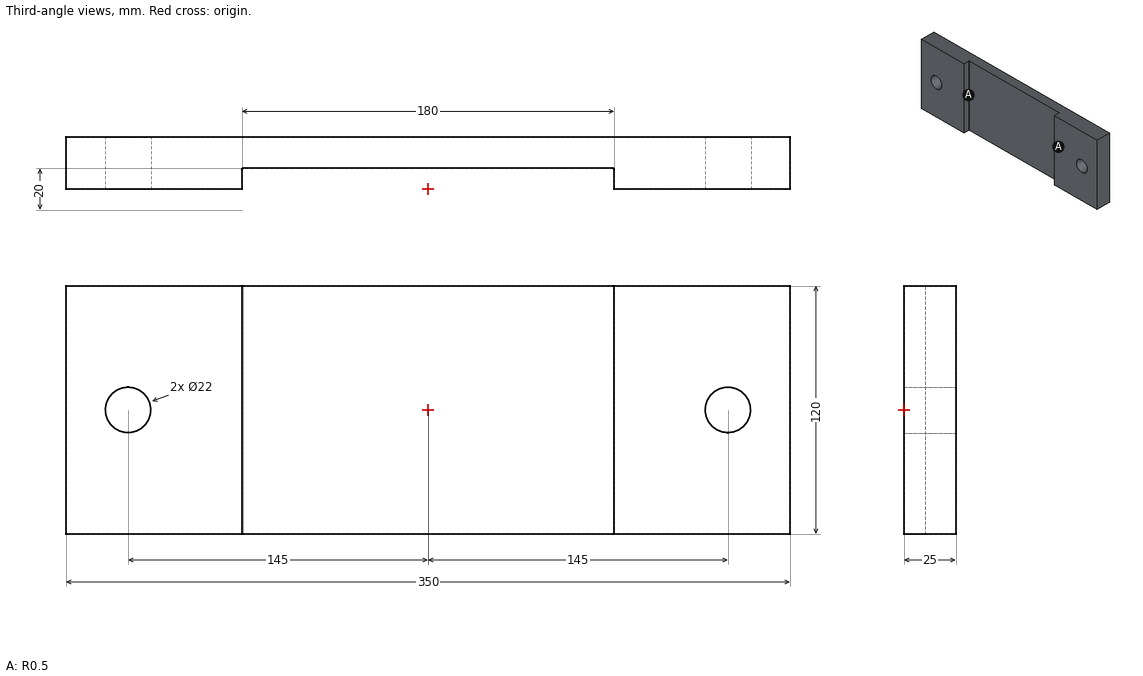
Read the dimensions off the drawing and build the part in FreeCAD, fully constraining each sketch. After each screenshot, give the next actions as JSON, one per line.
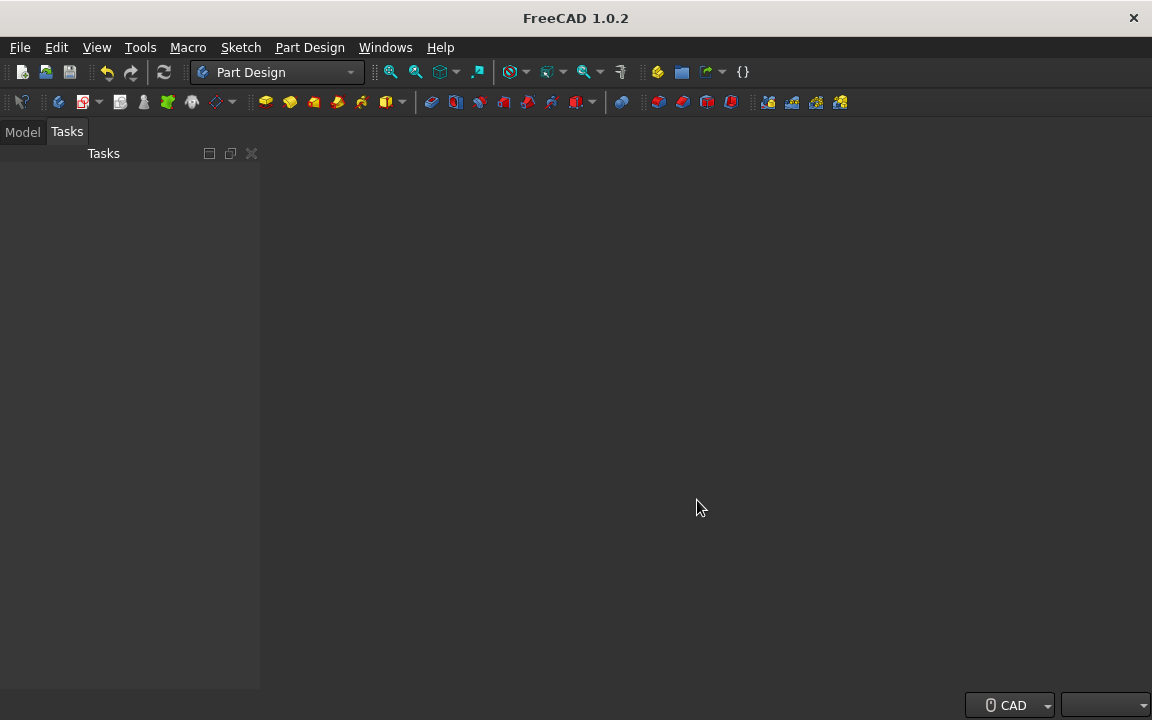
{"action": "left_click", "coordinate": [22, 72]}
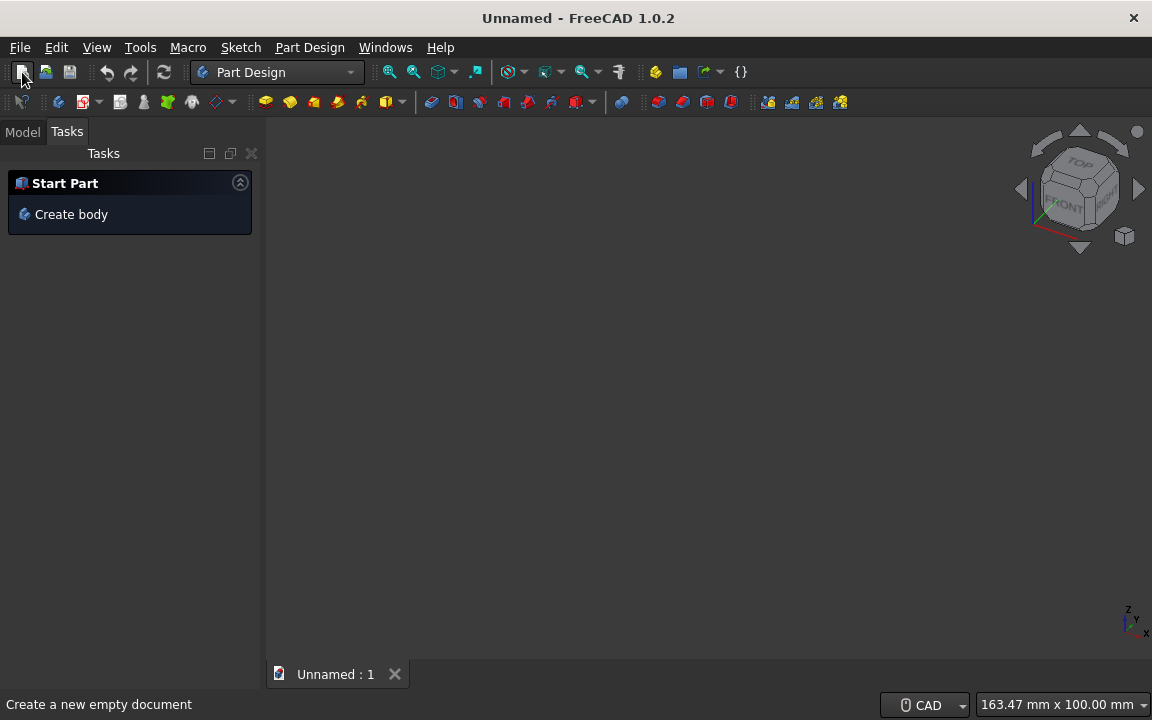
{"action": "left_click", "coordinate": [84, 102]}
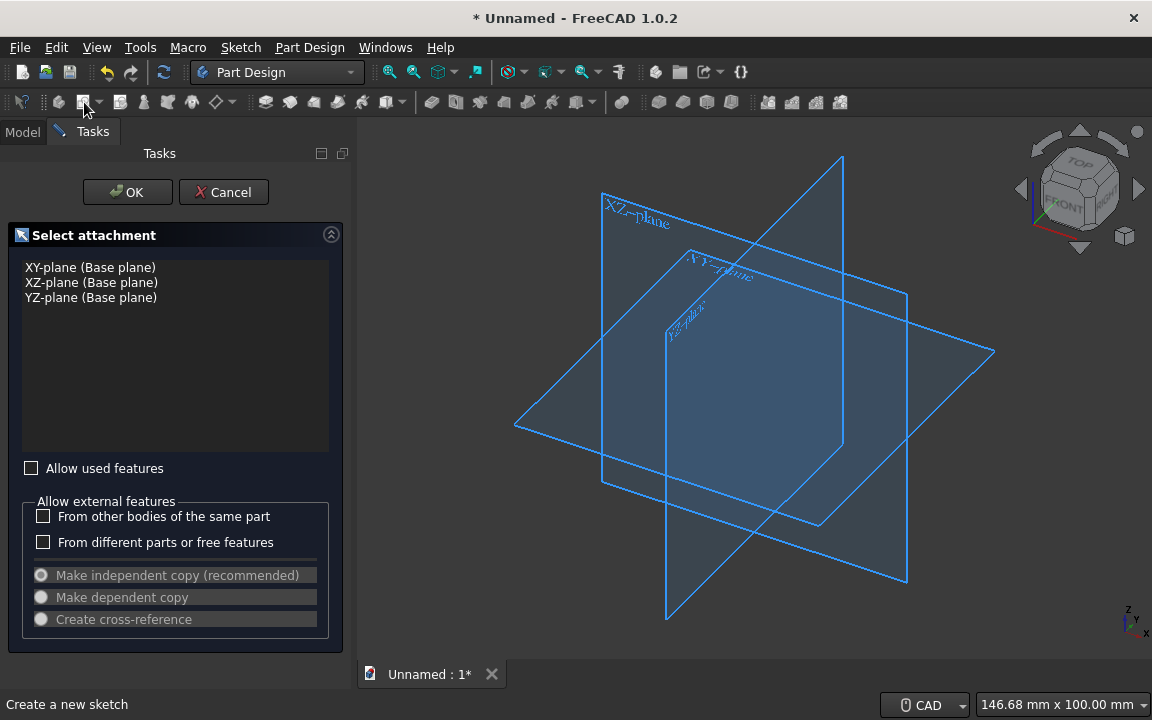
{"action": "left_click", "coordinate": [82, 282]}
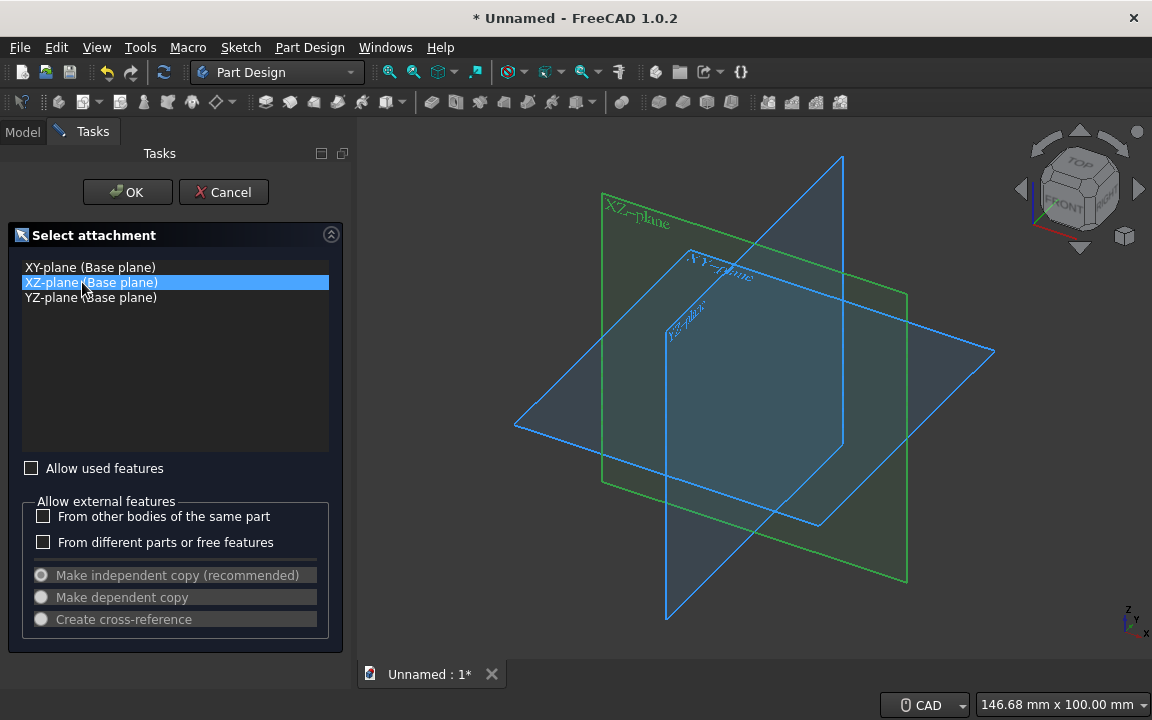
{"action": "left_click", "coordinate": [128, 192]}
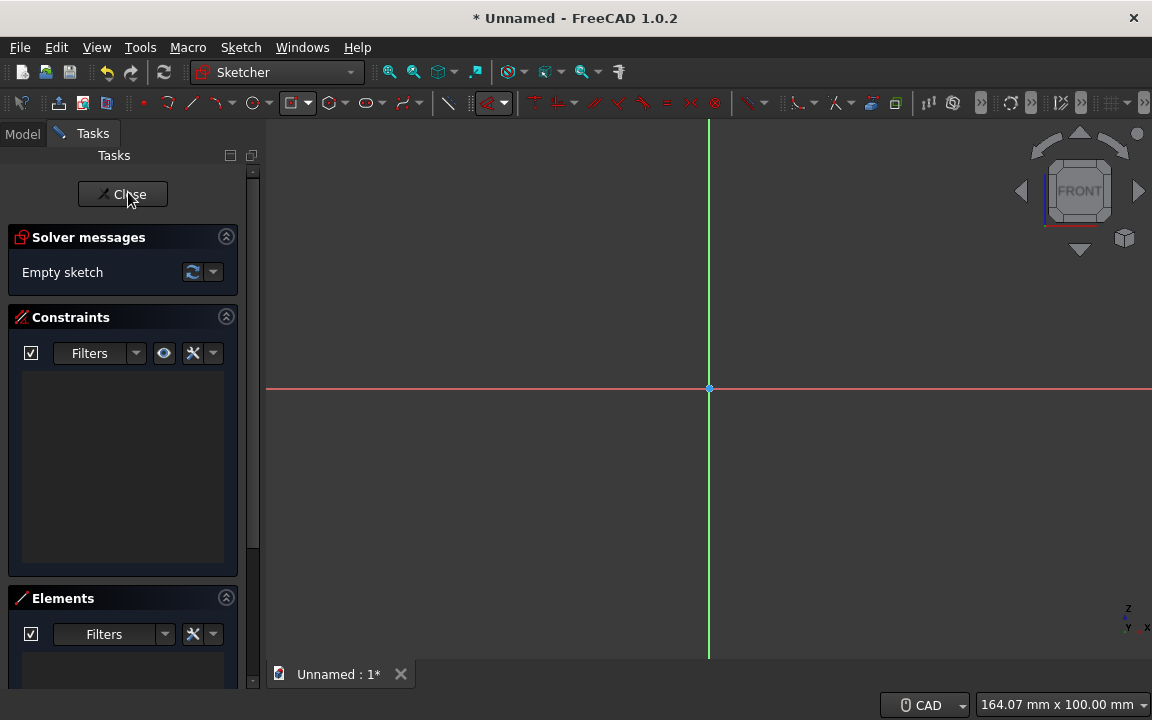
{"action": "scroll", "coordinate": [618, 389], "scroll_direction": "down", "scroll_amount": 7}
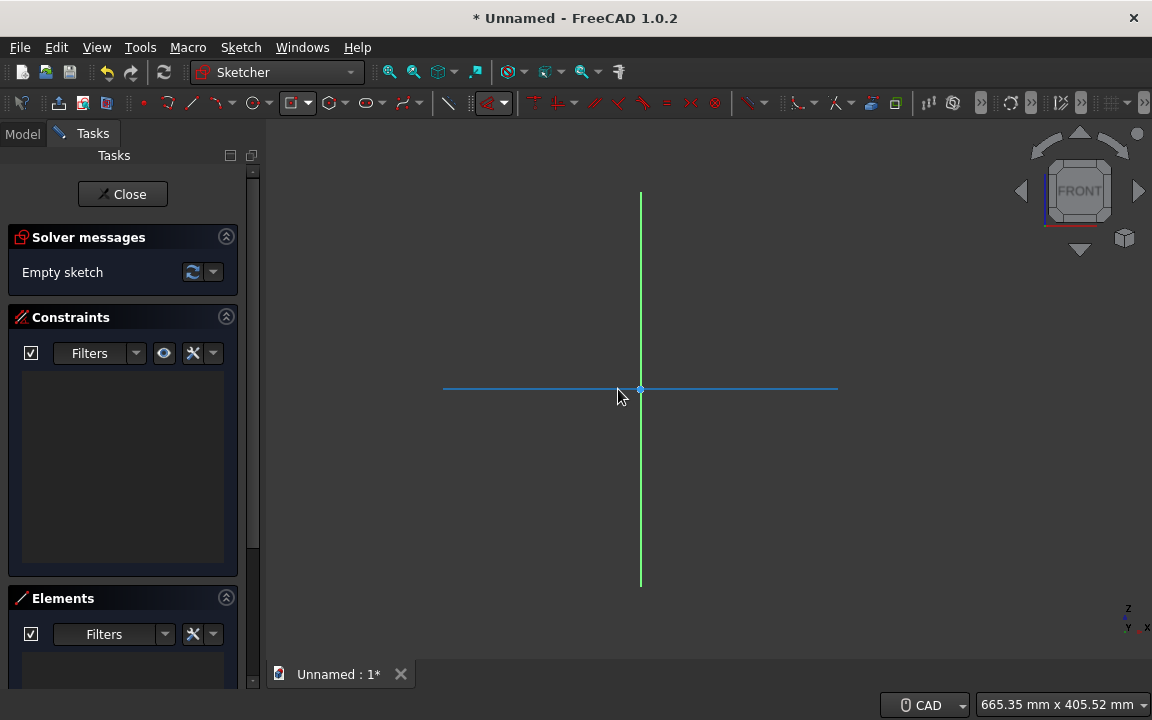
{"action": "left_click", "coordinate": [292, 104]}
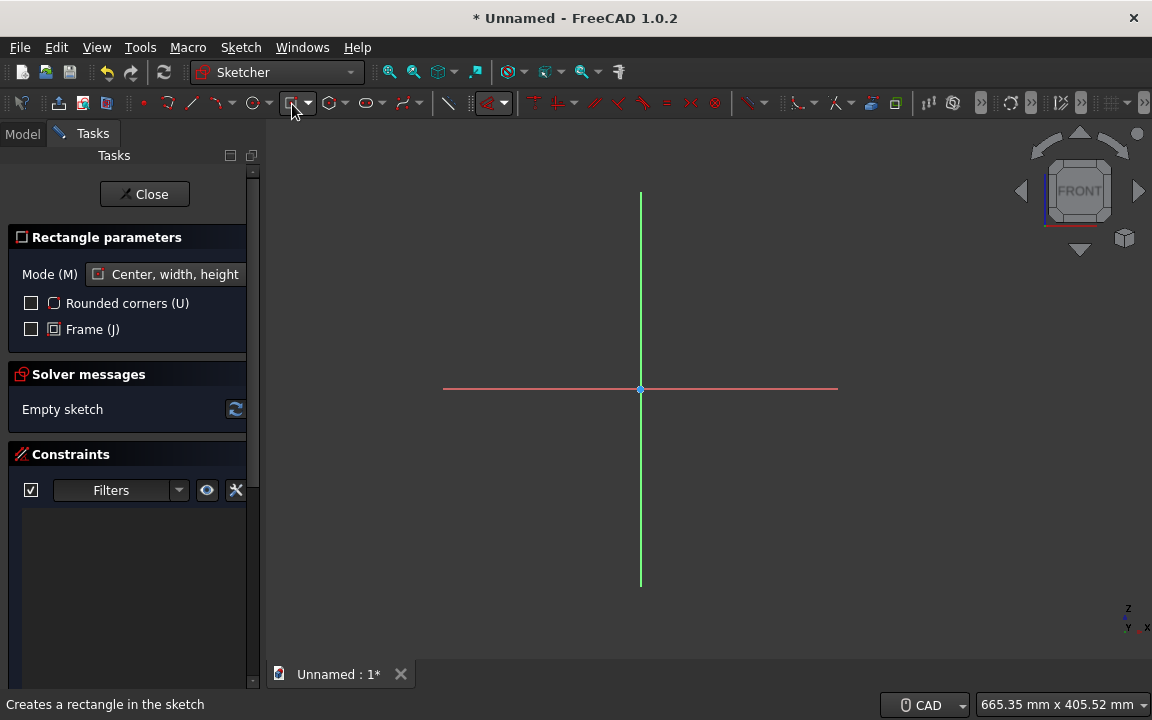
{"action": "left_click", "coordinate": [641, 389]}
{"action": "mouse_move", "coordinate": [874, 309]}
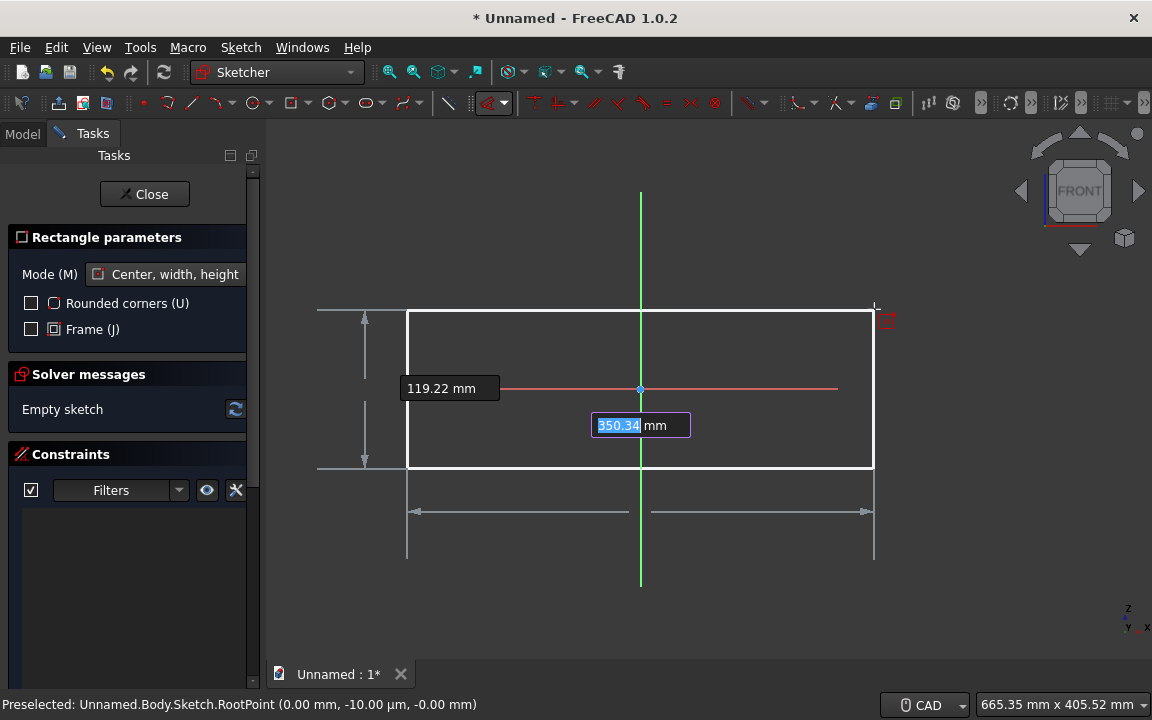
{"action": "type", "text": "350"}
{"action": "key", "text": "Tab"}
{"action": "type", "text": "120"}
{"action": "key", "text": "Return"}
{"action": "key", "text": "Escape"}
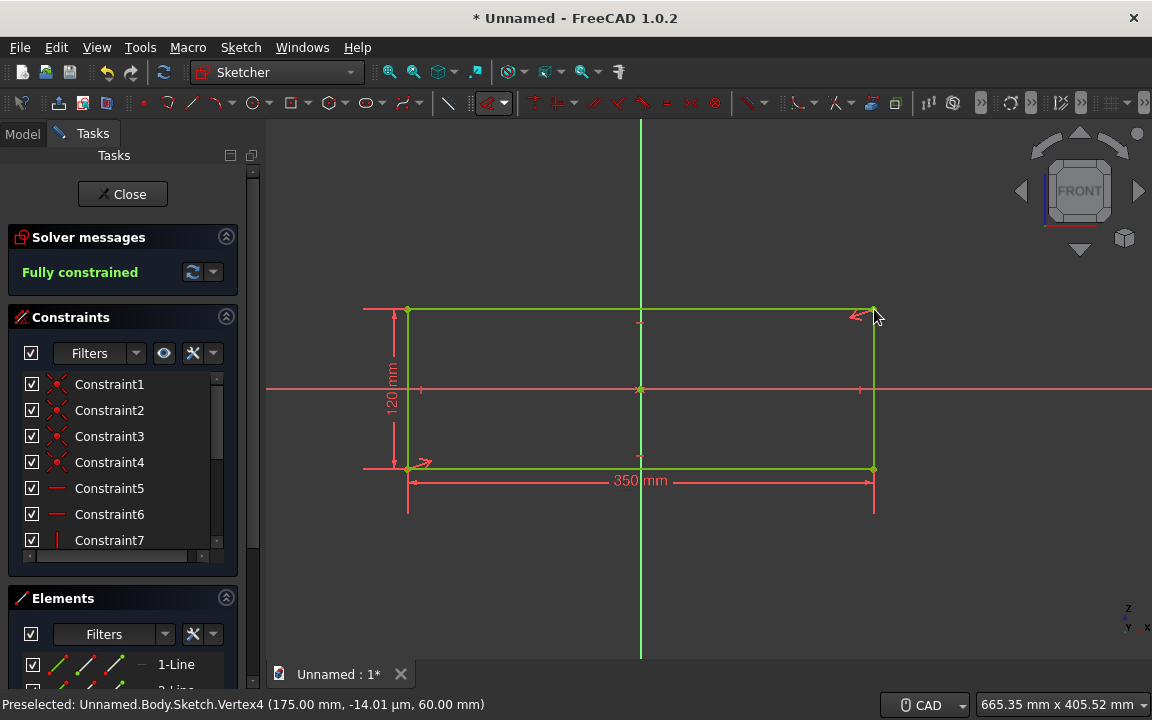
{"action": "left_click", "coordinate": [123, 194]}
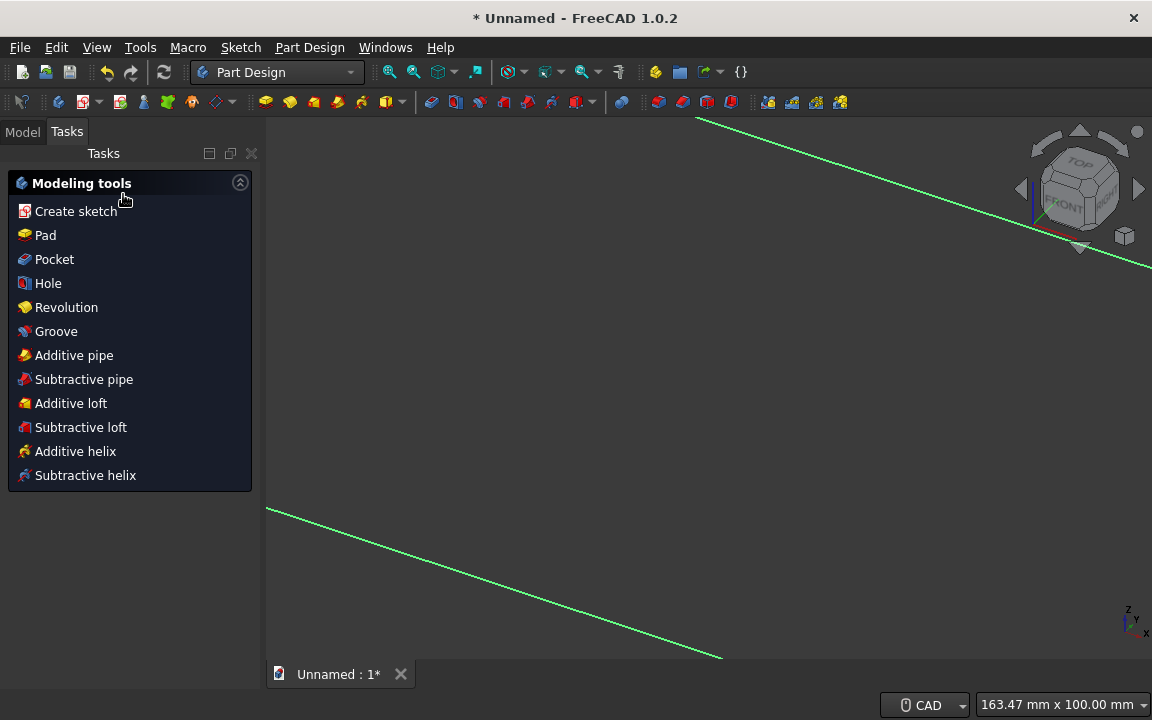
{"action": "left_click", "coordinate": [266, 102]}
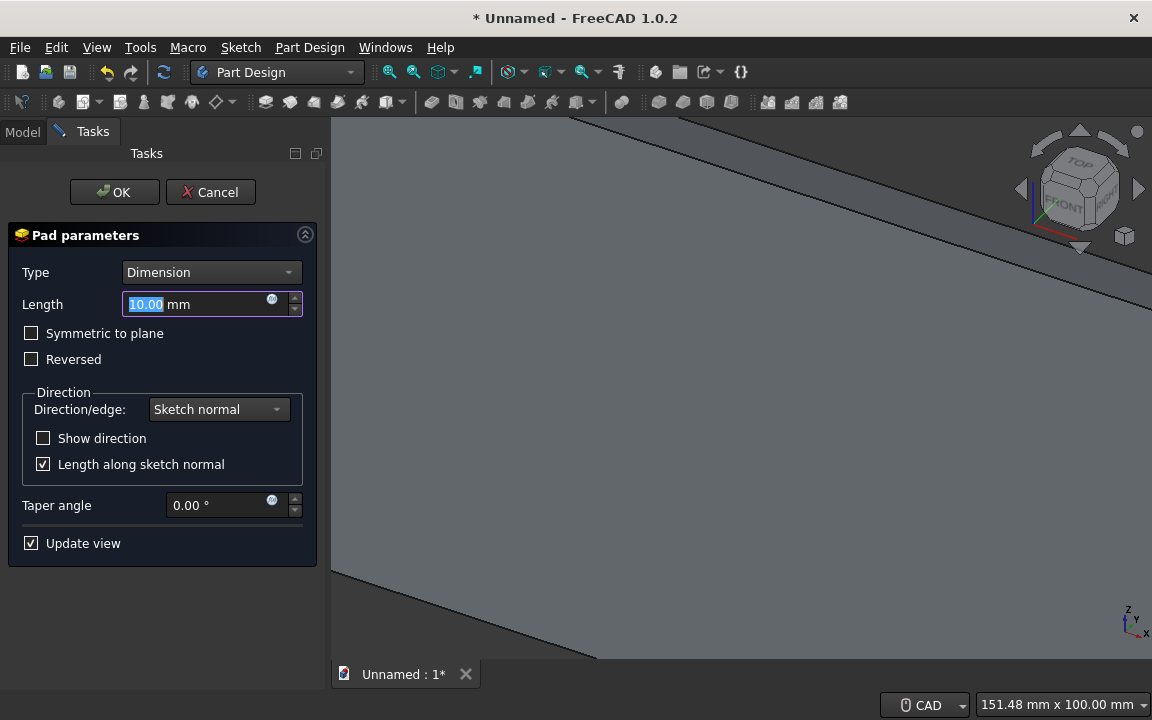
{"action": "type", "text": "25"}
{"action": "key", "text": "Tab"}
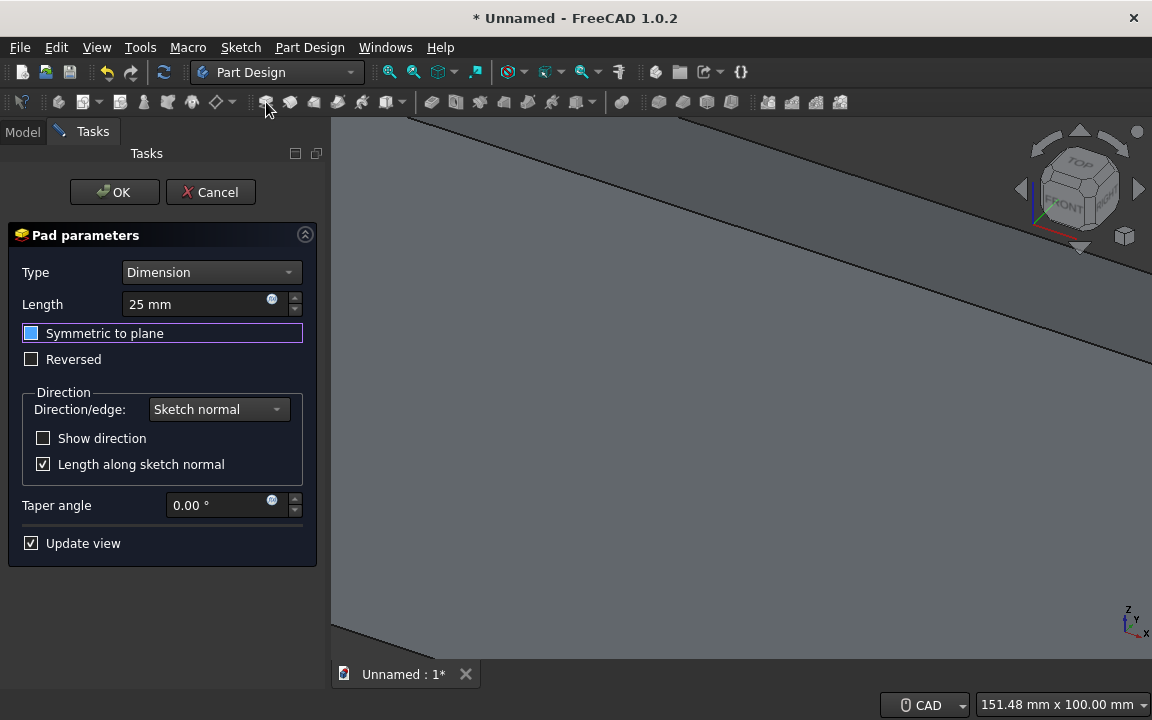
{"action": "left_click", "coordinate": [30, 359]}